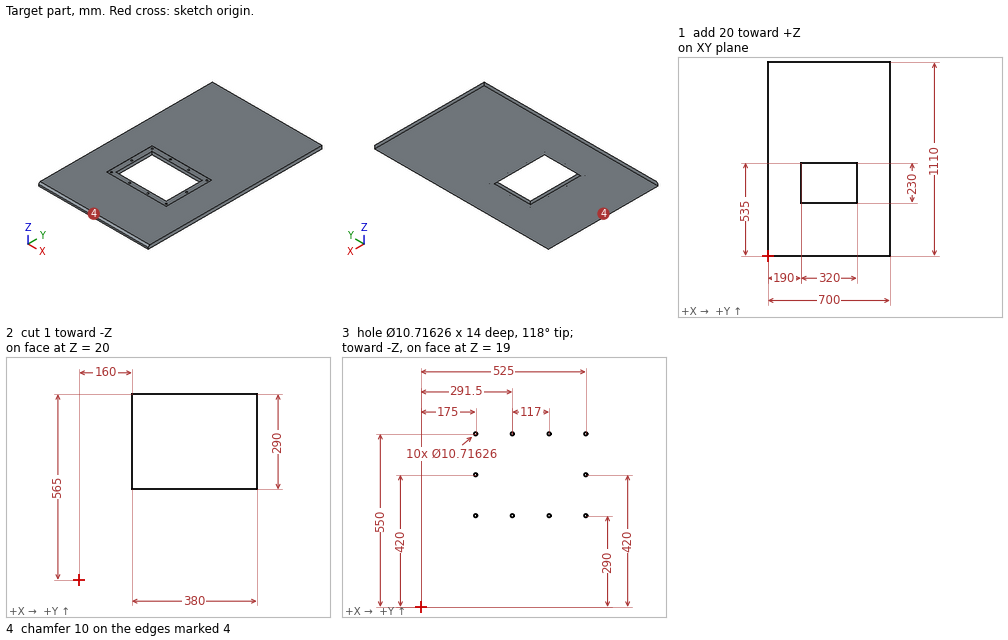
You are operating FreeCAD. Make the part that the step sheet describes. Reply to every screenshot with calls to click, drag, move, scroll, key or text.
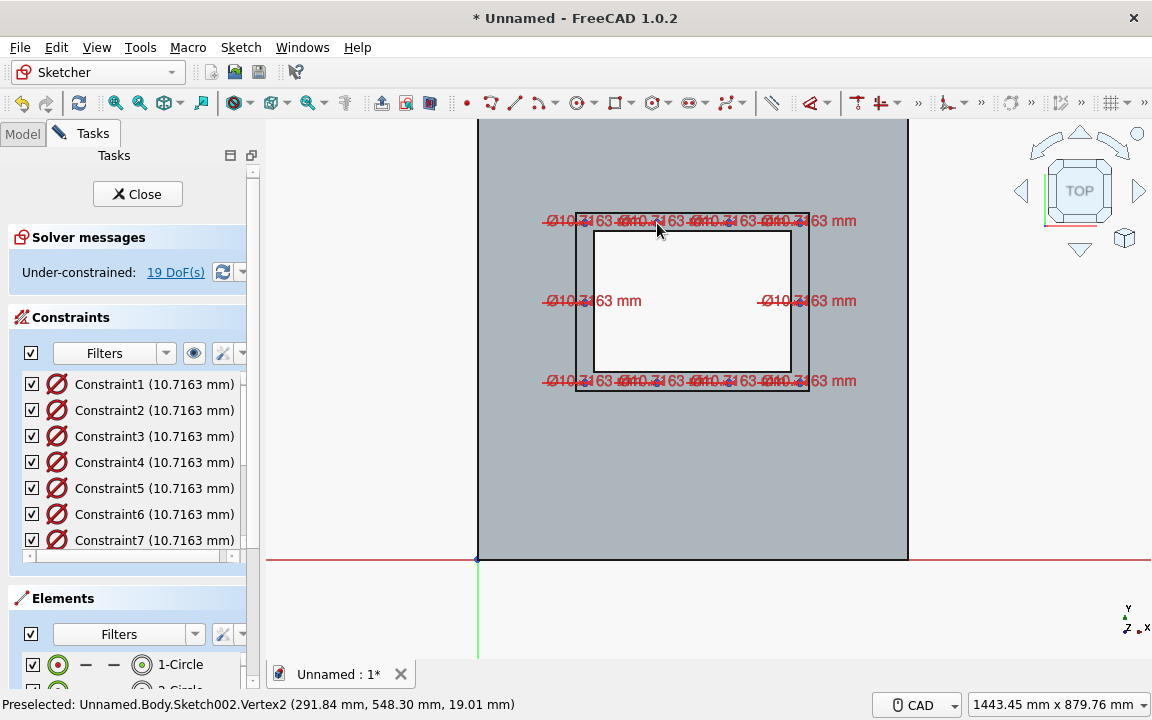
click(657, 223)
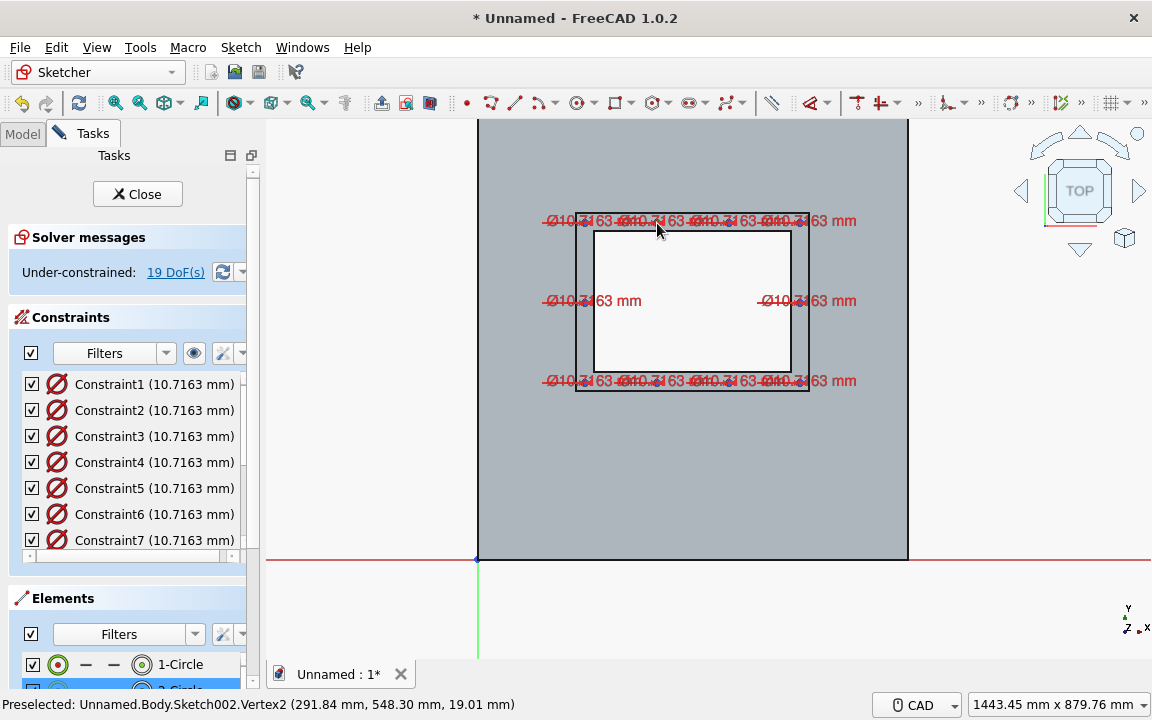
click(729, 223)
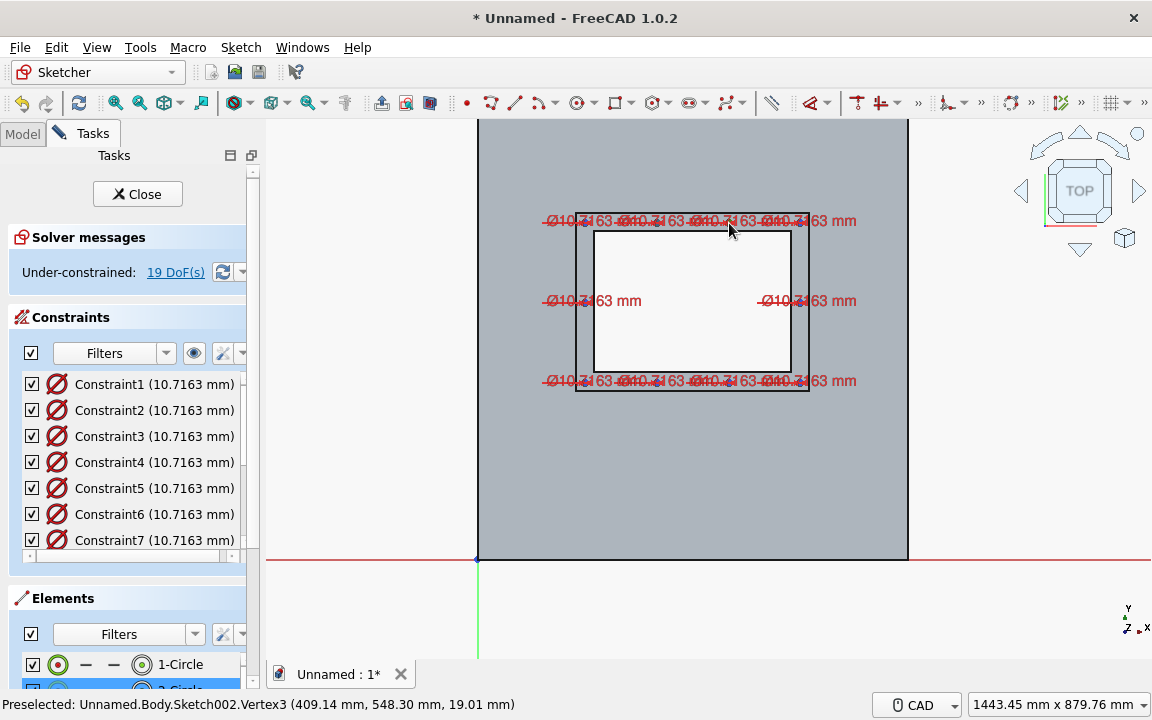
click(900, 104)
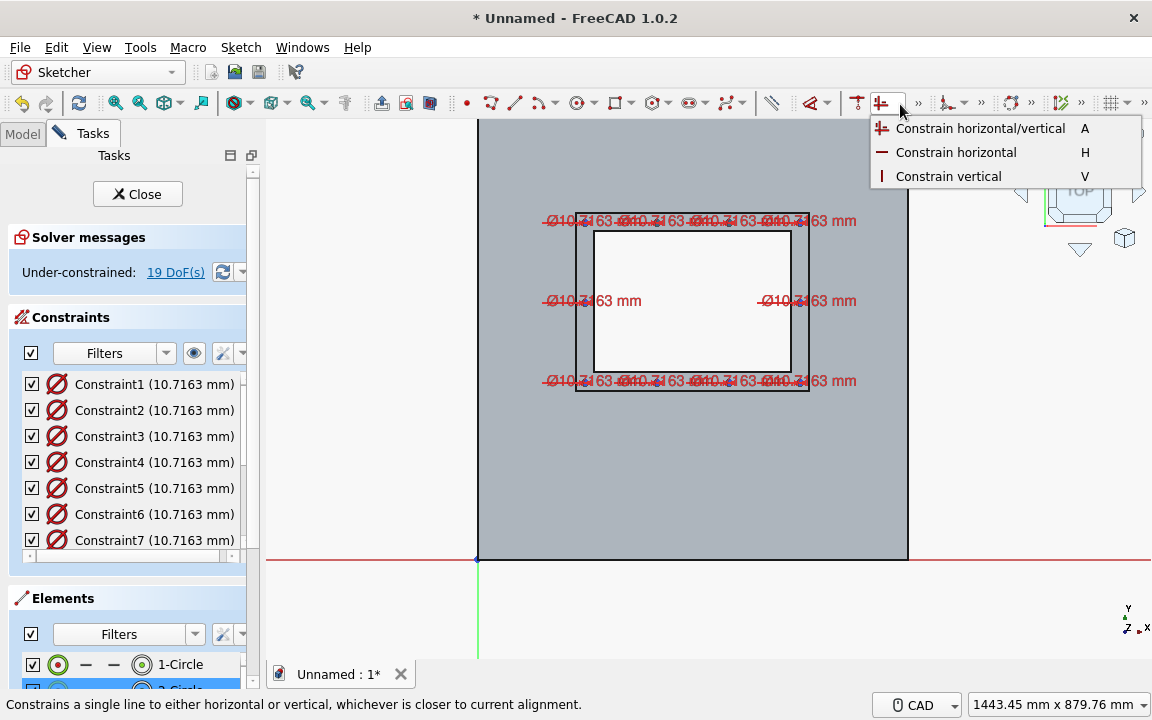
click(1006, 152)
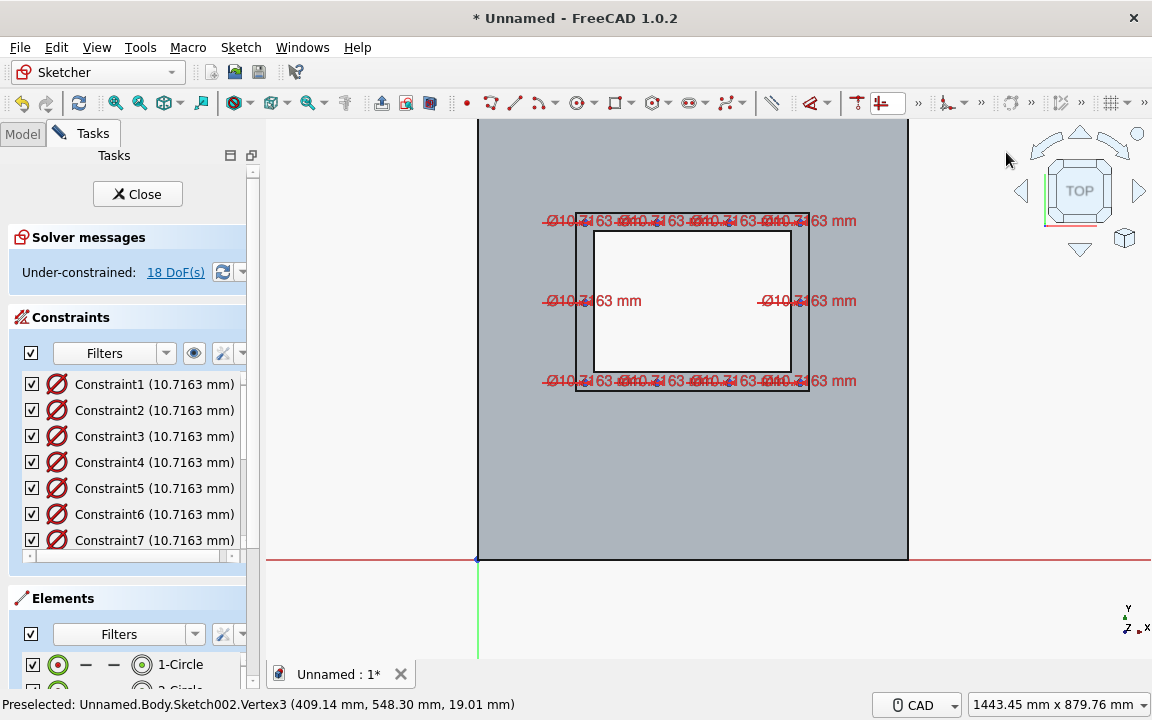
click(729, 223)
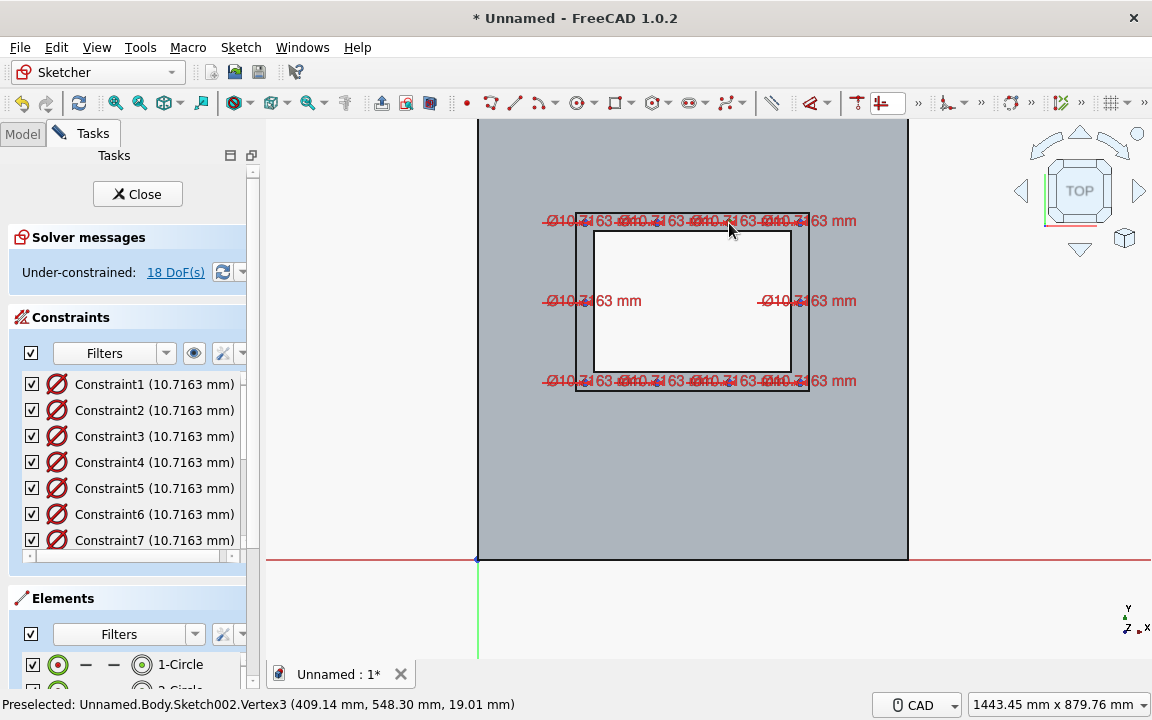
click(800, 223)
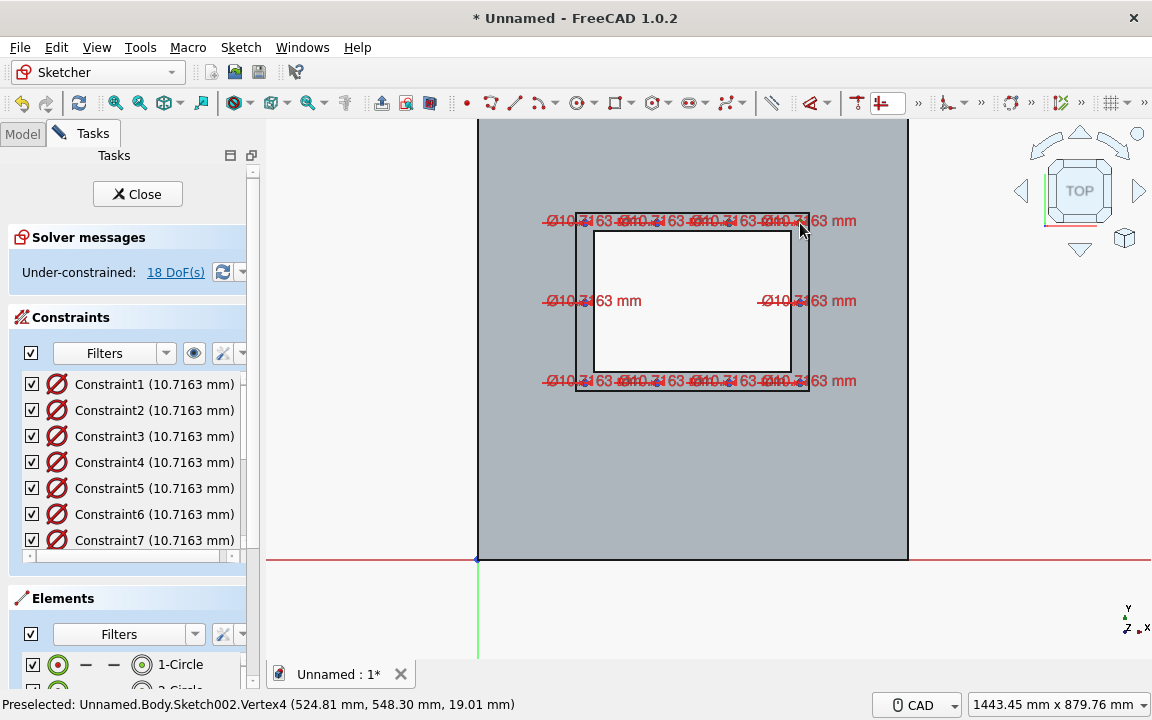
key(h)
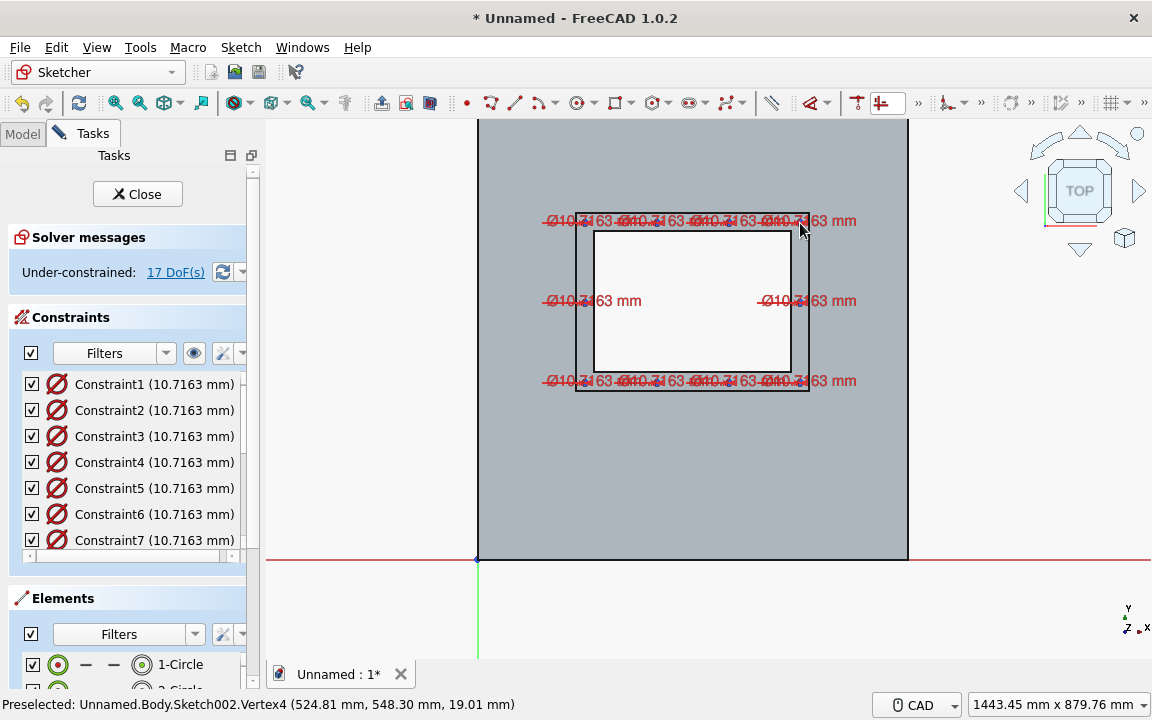
click(800, 223)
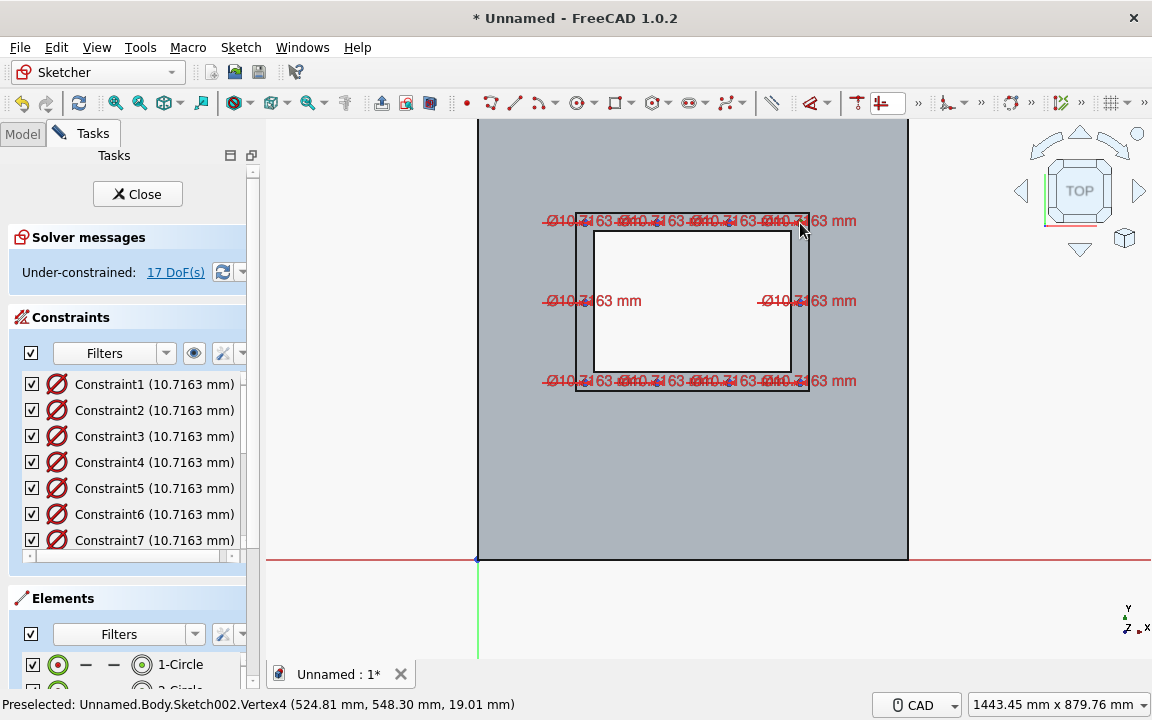
click(800, 303)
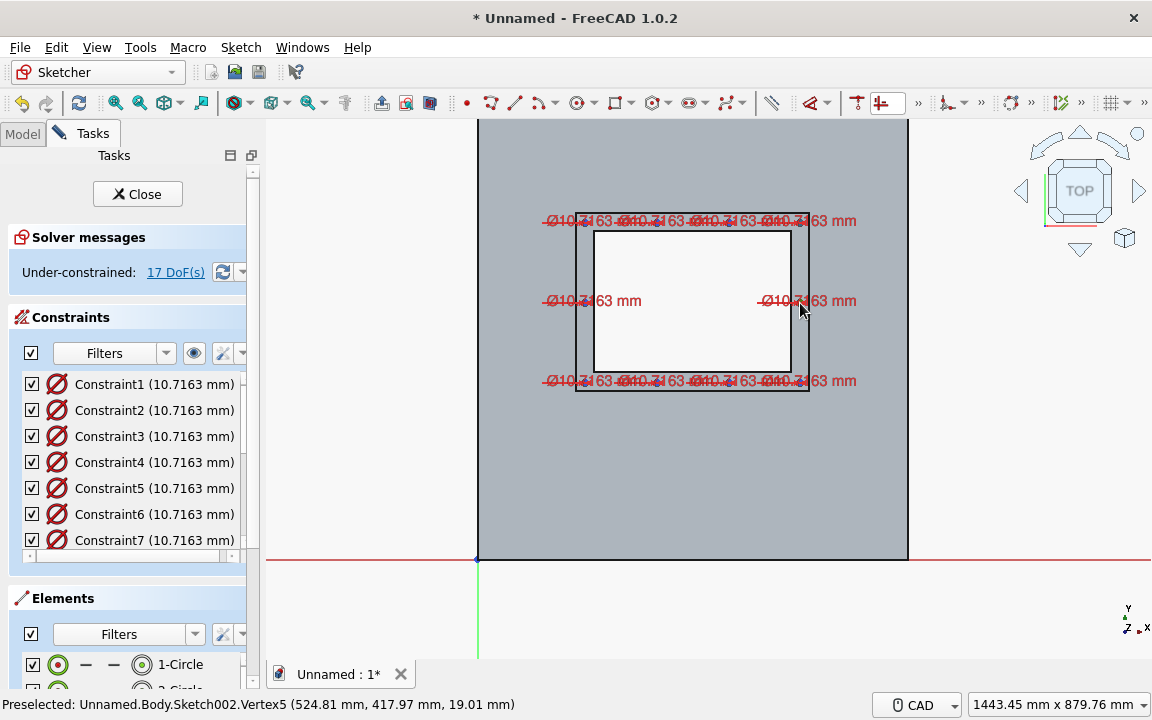
key(v)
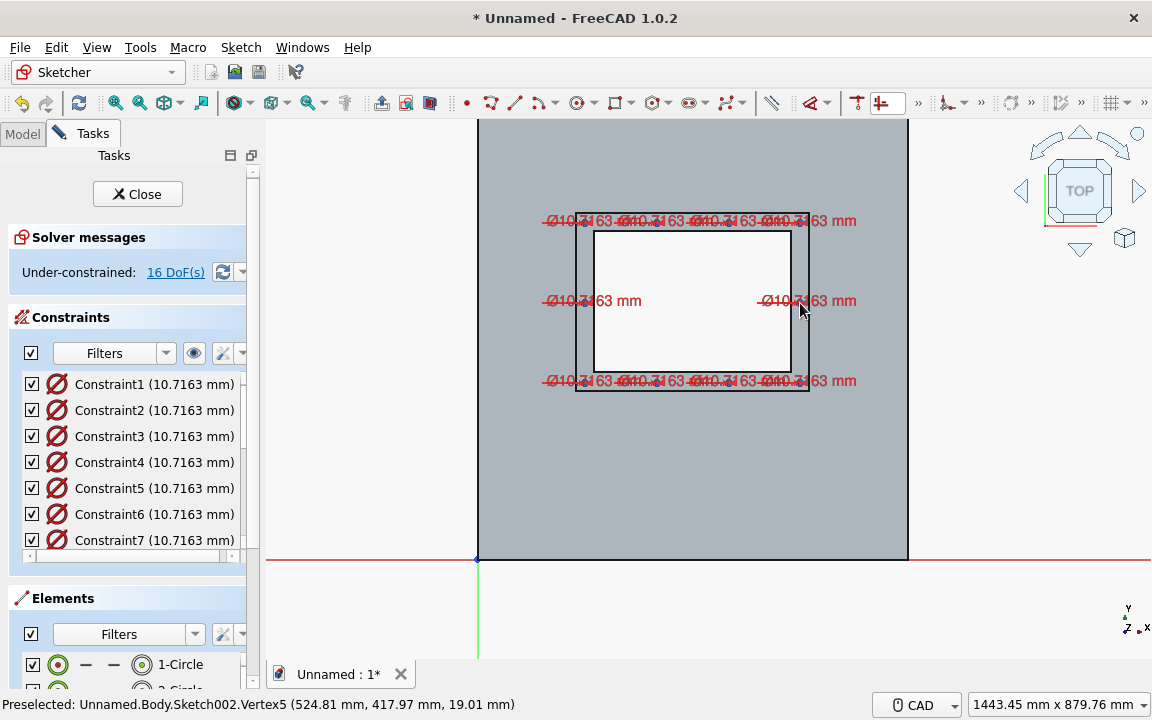
click(800, 303)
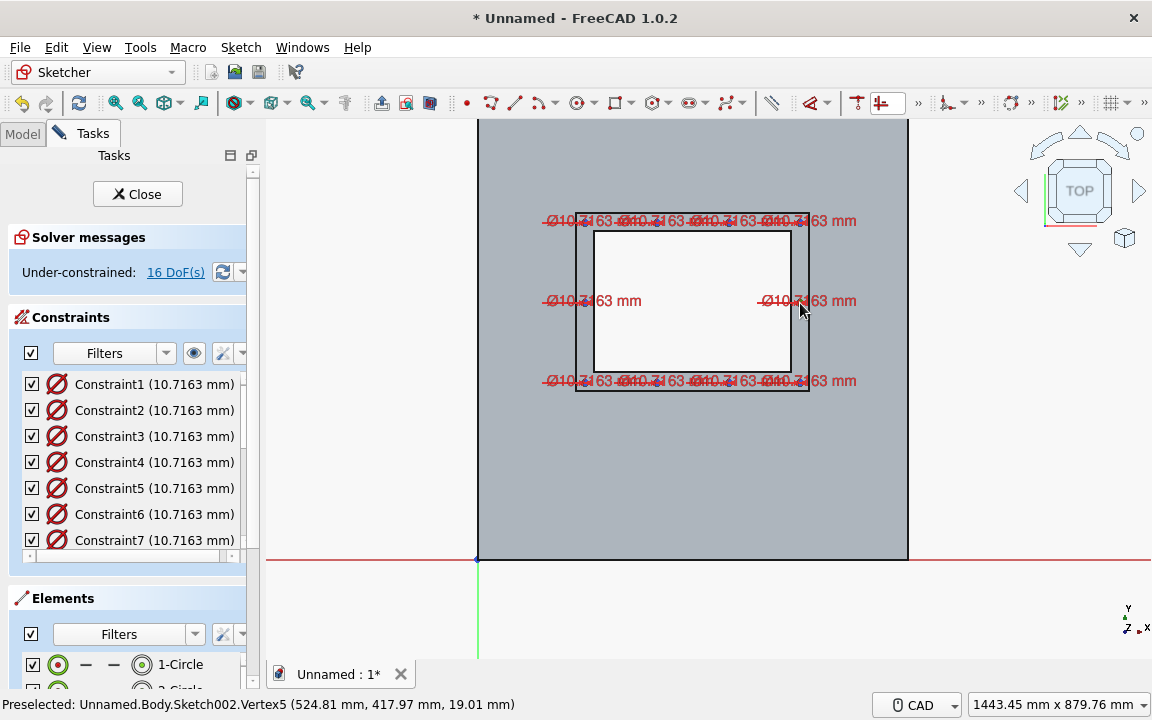
click(800, 383)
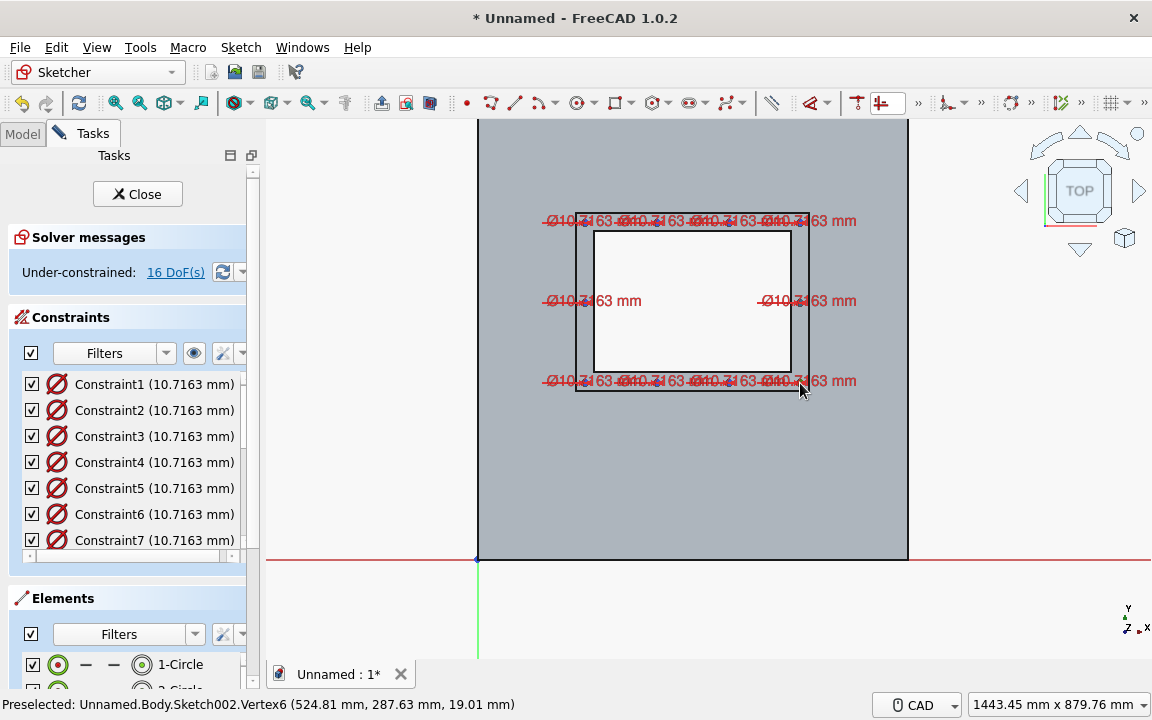
key(v)